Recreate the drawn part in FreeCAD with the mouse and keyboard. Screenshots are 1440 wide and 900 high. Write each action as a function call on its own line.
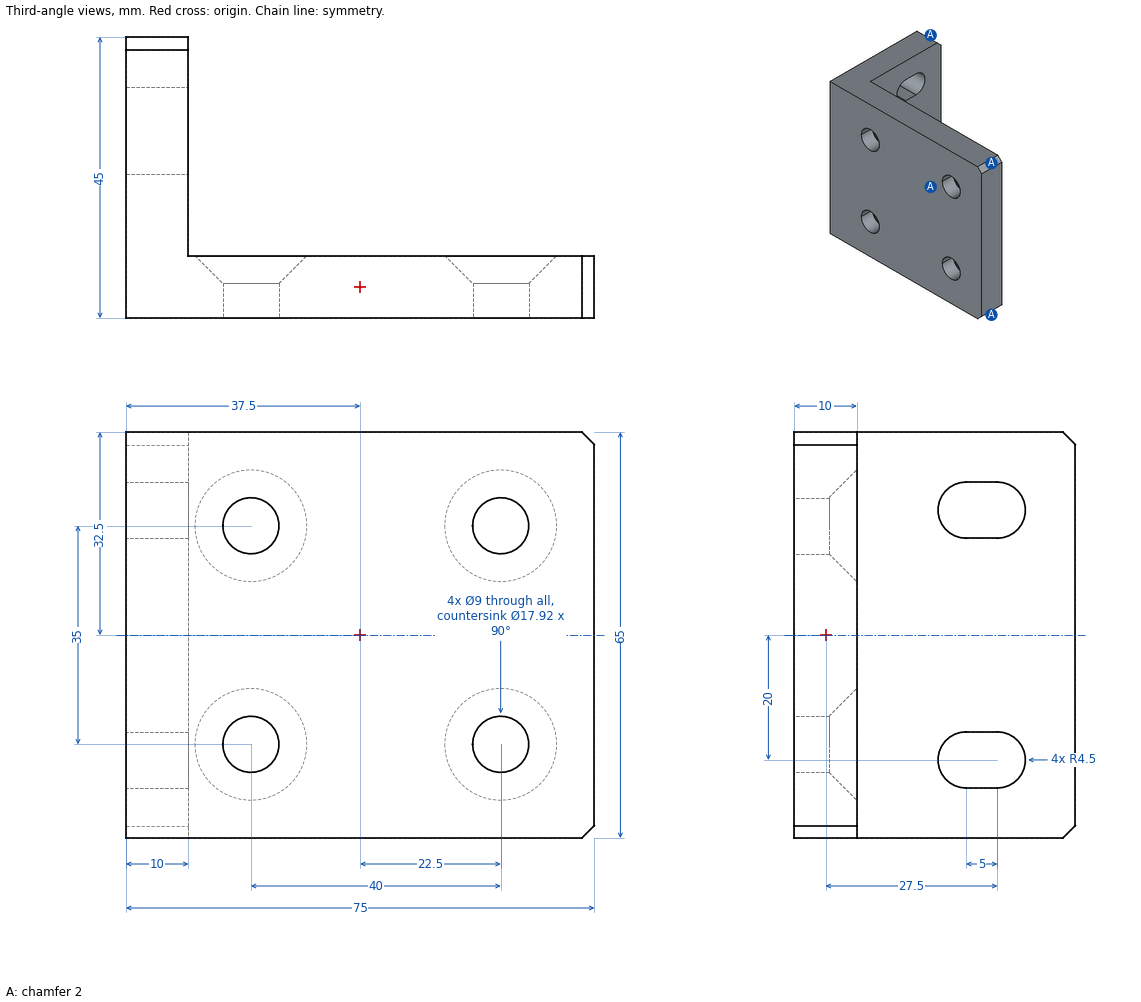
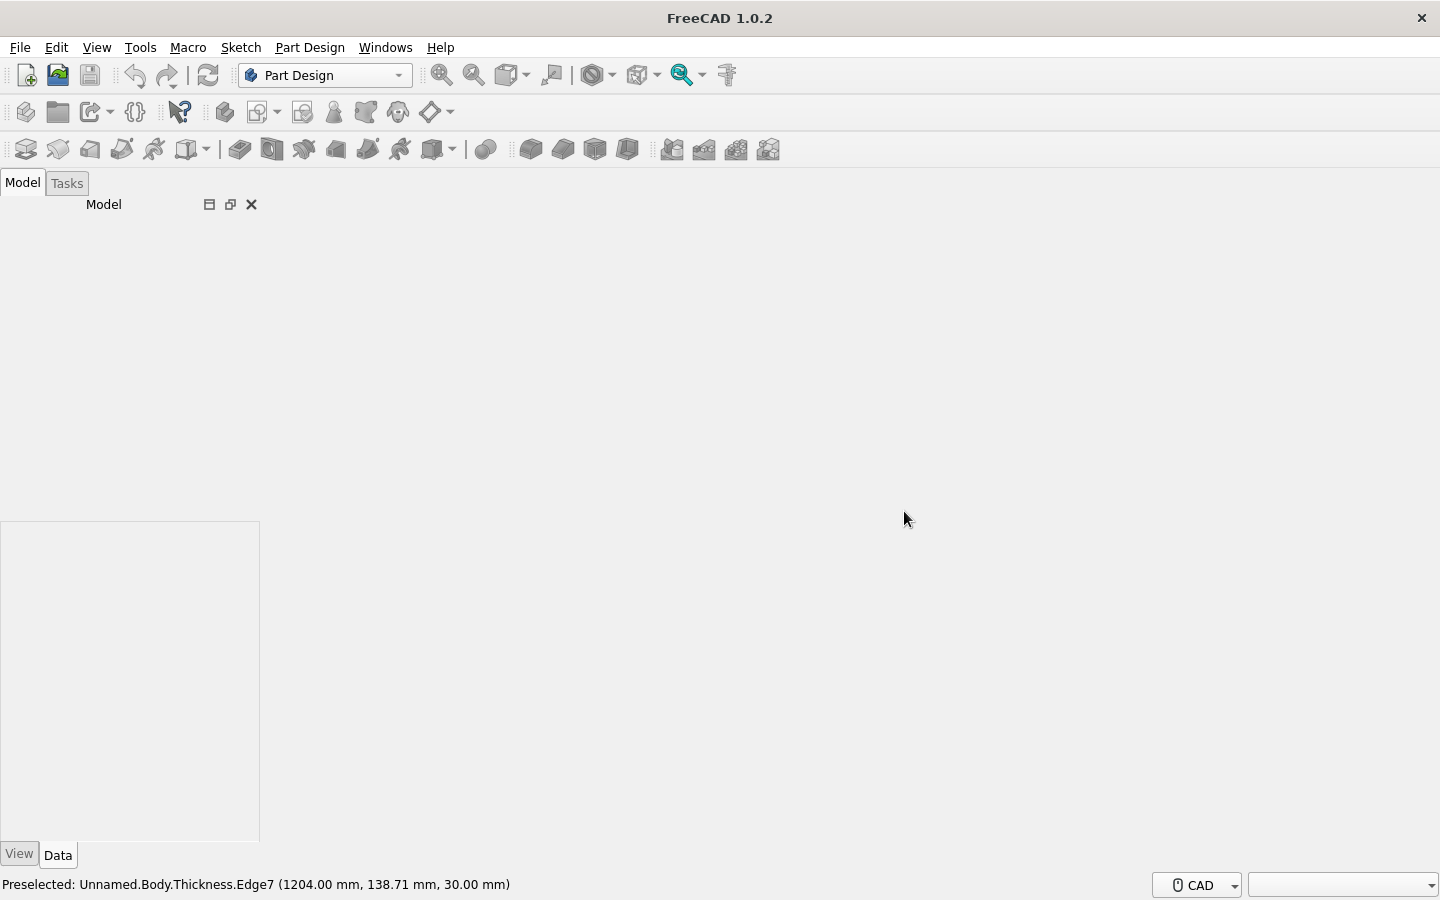
key(ctrl+n)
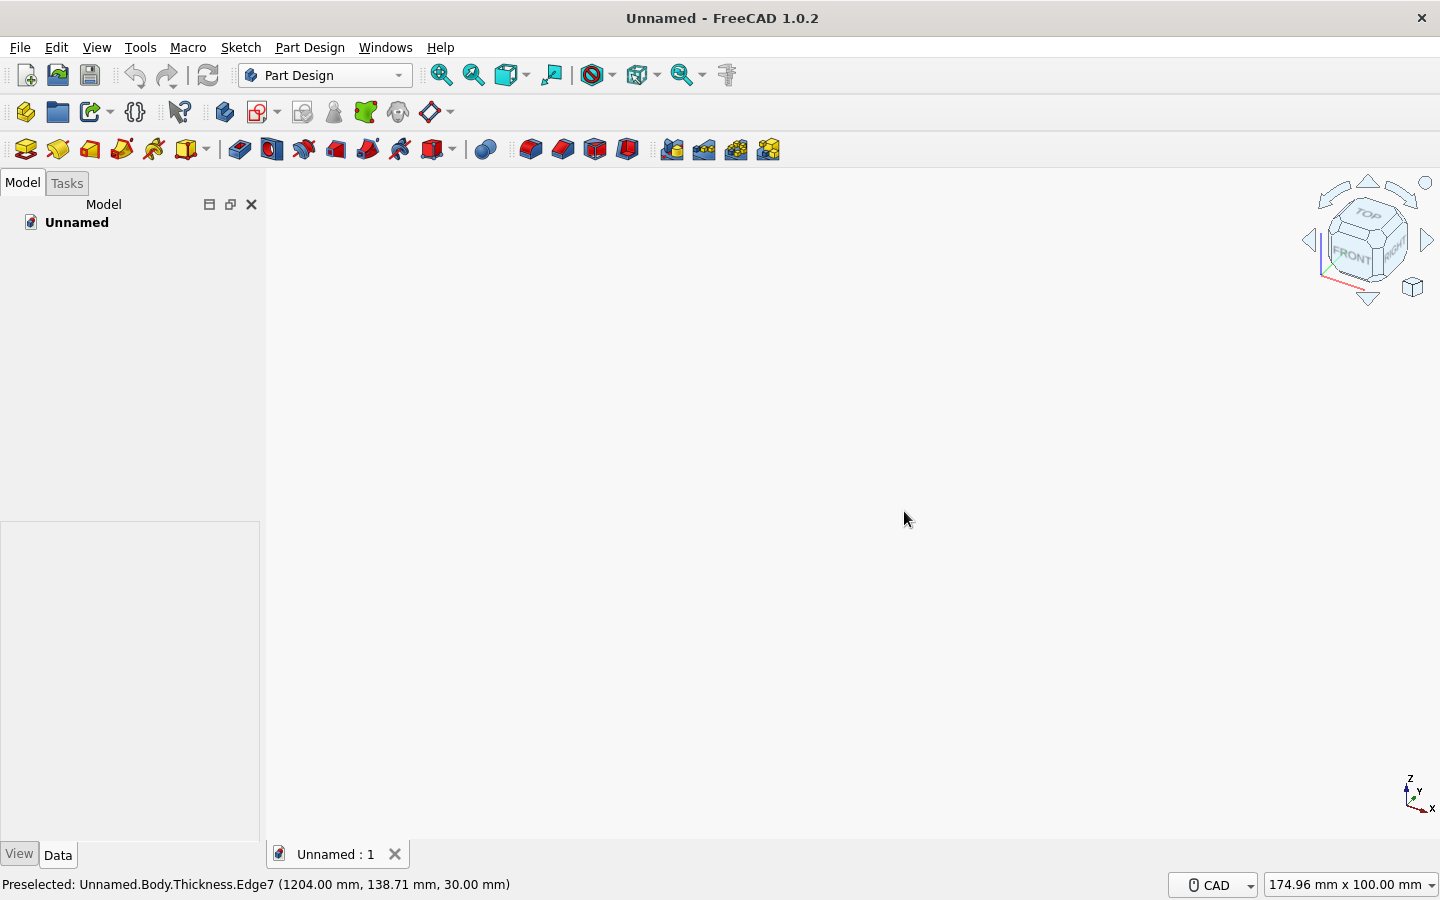
click(258, 112)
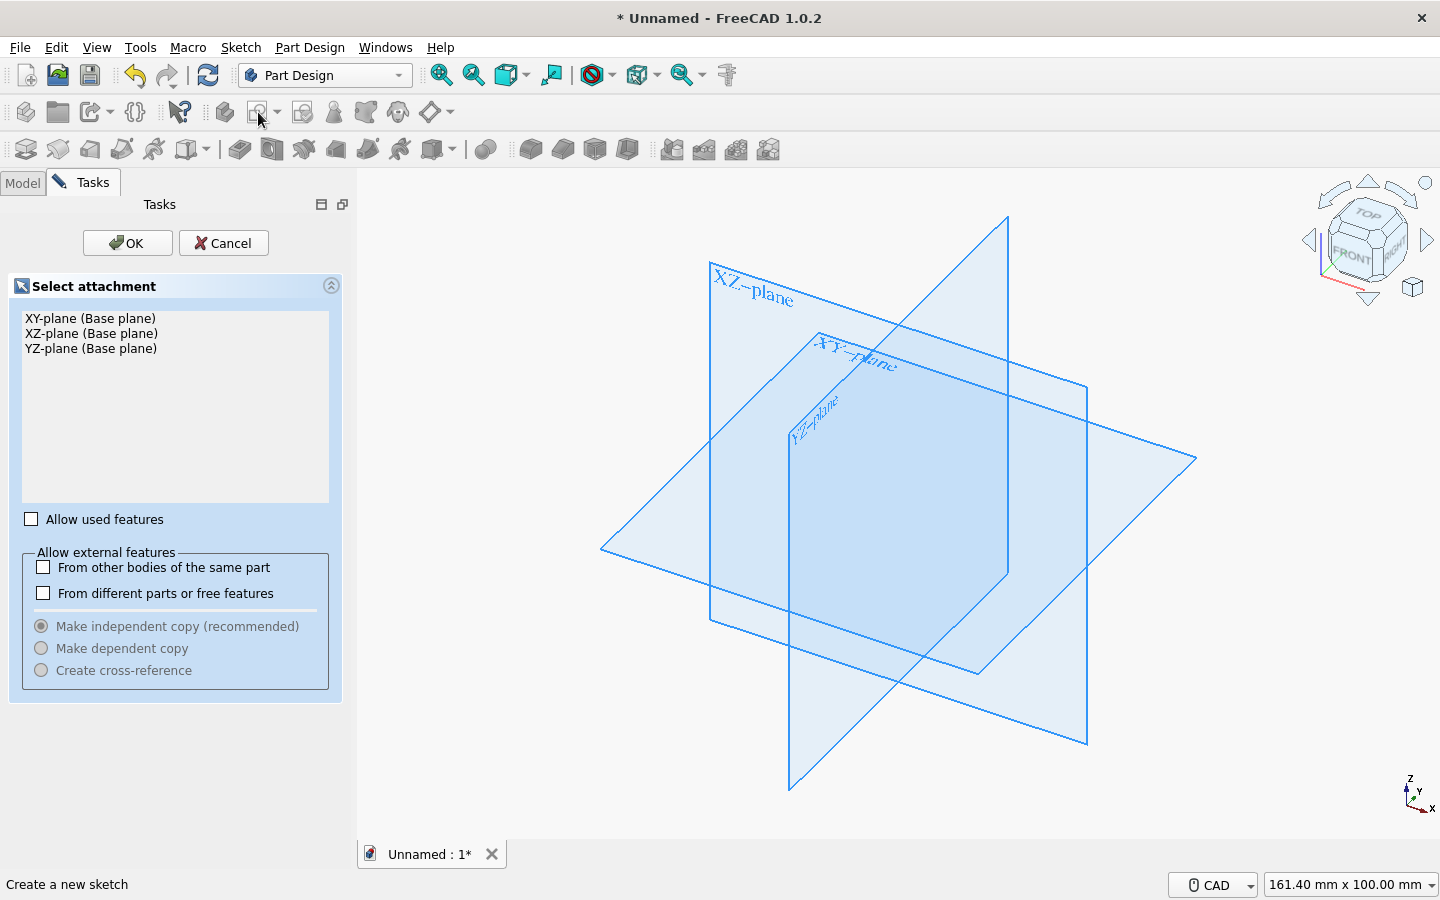
click(82, 334)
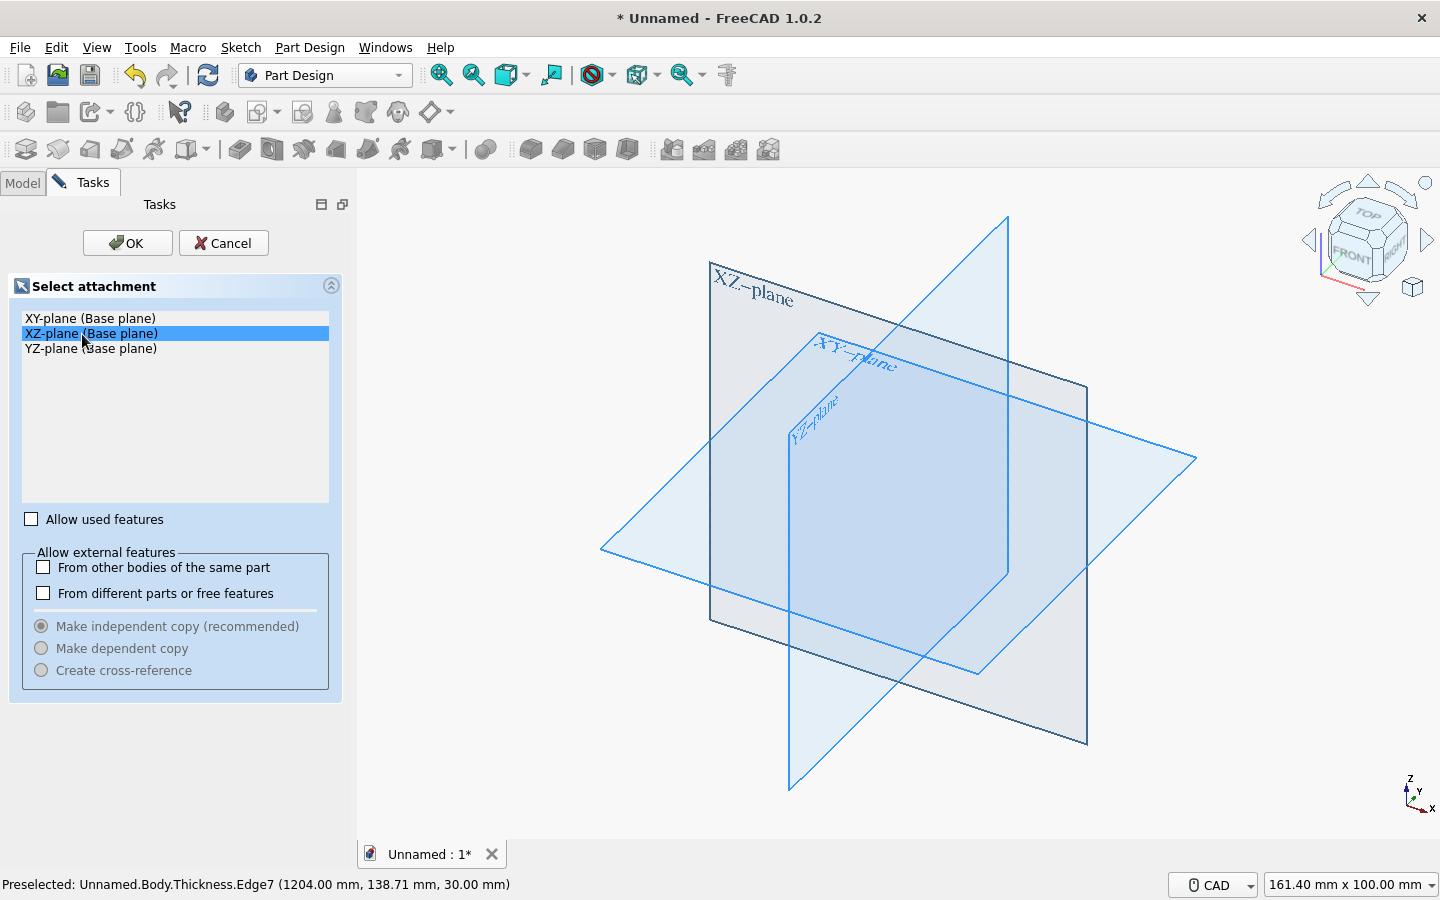
click(128, 243)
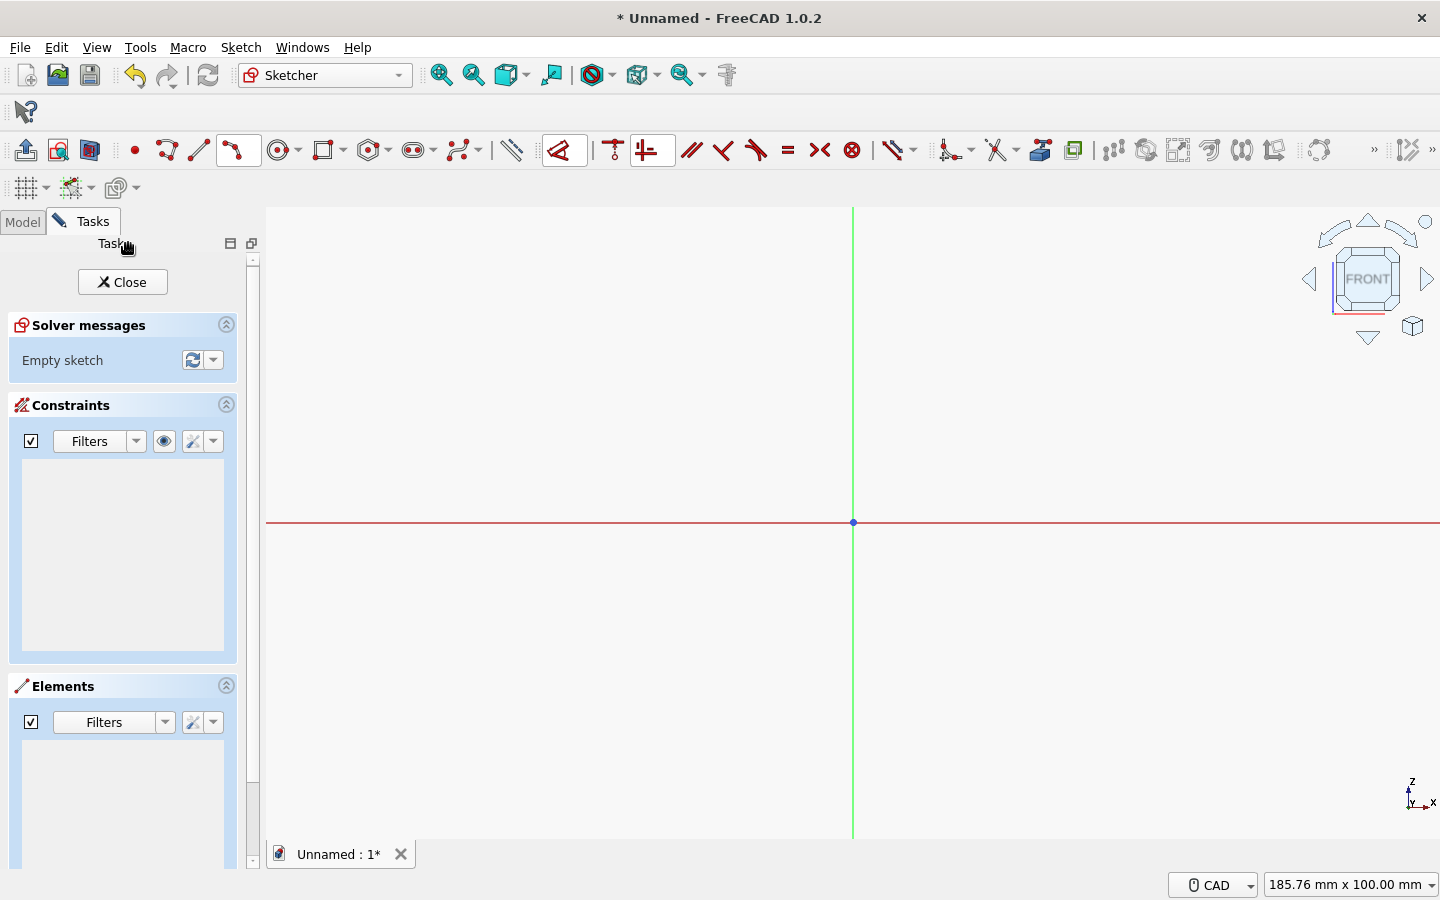
key(g)
key(v)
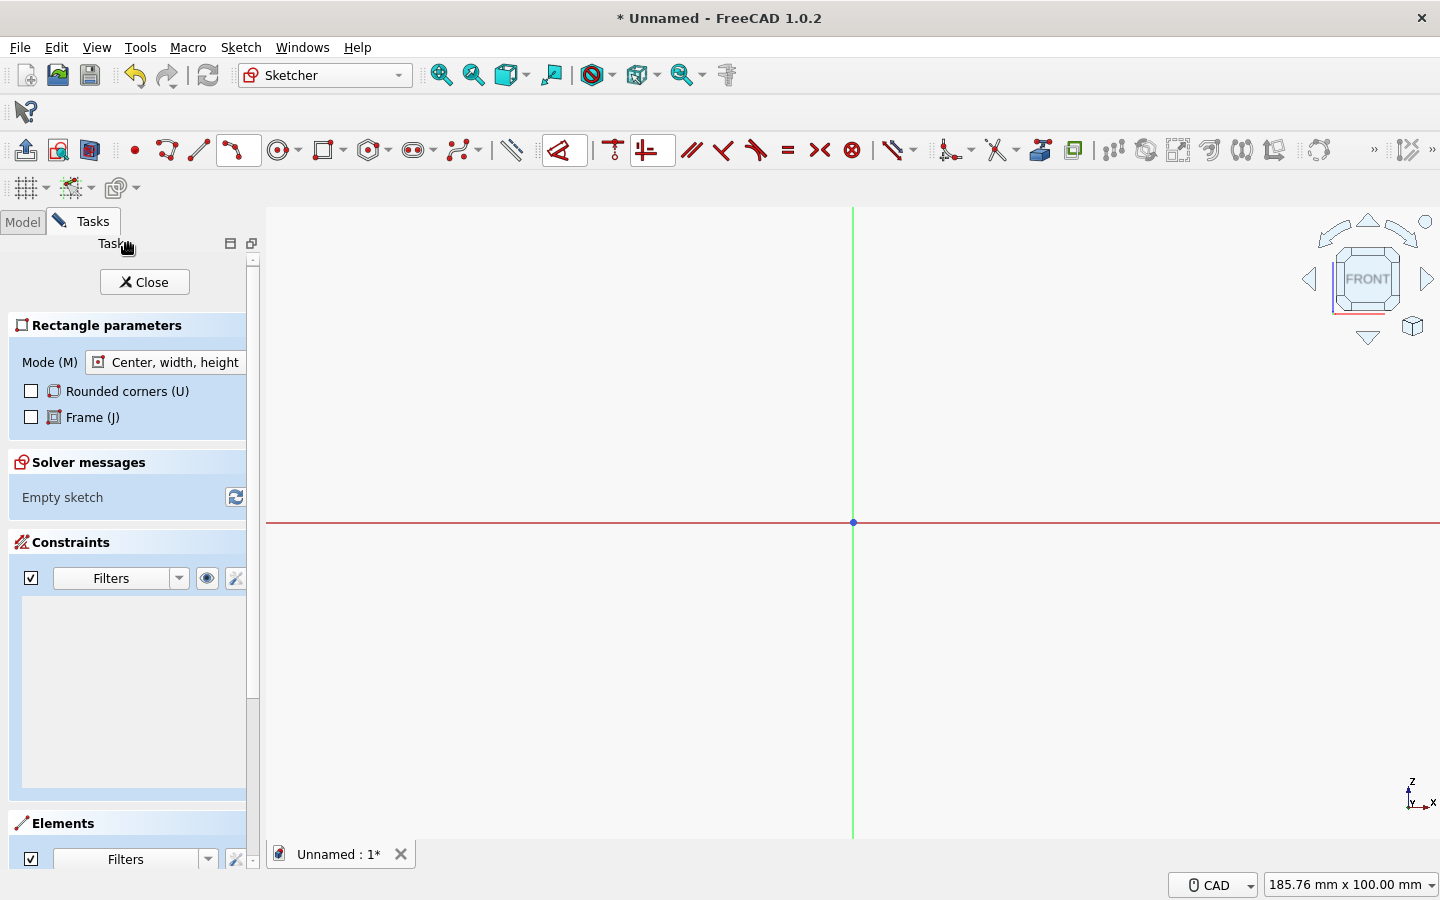
click(853, 523)
move(1090, 318)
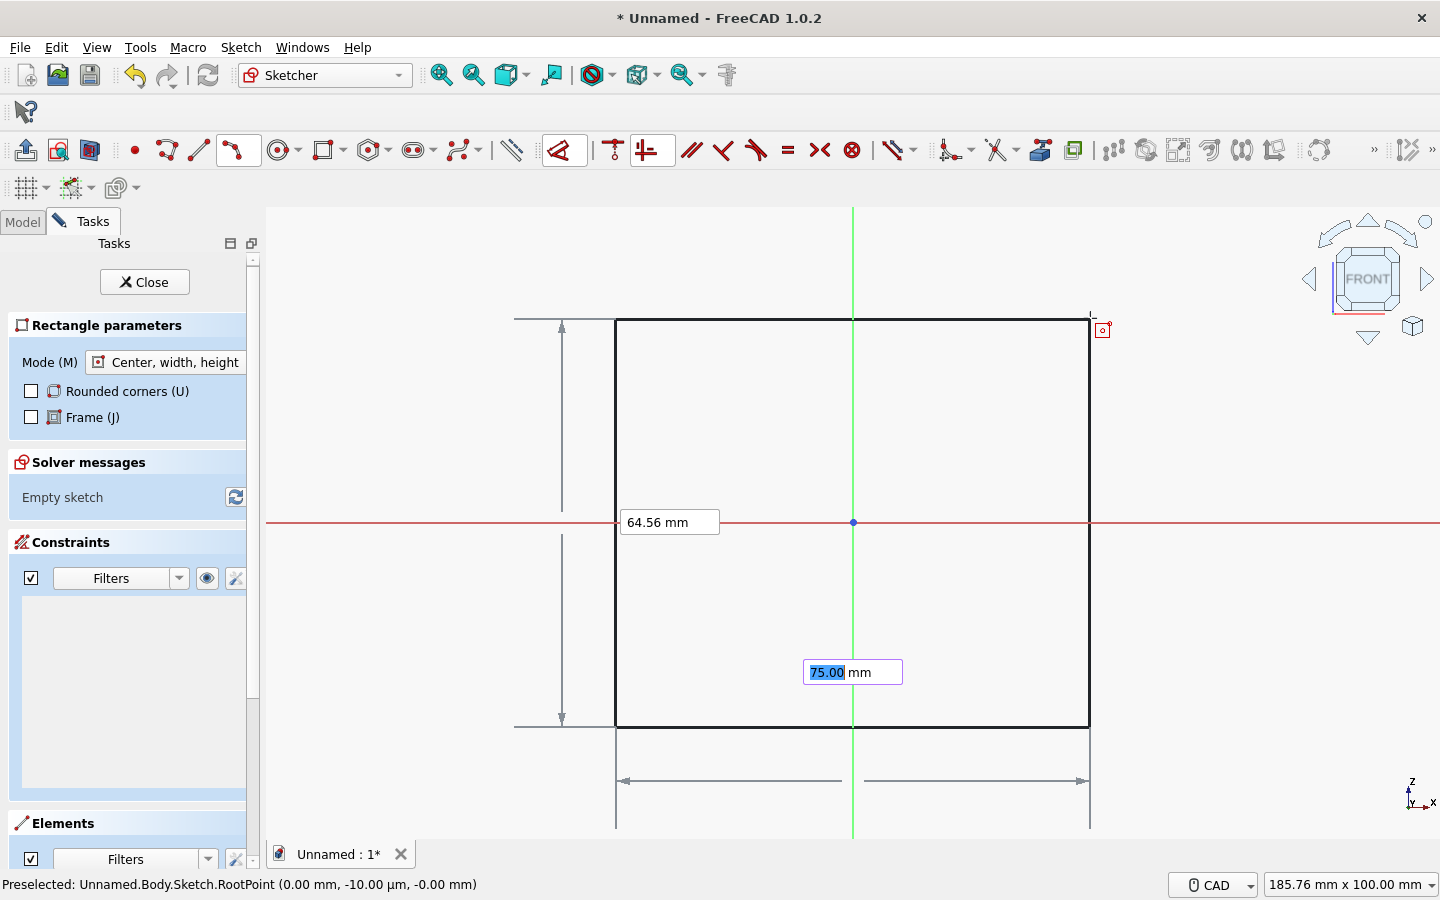
text(75)
key(Tab)
text(65)
key(Return)
key(Escape)